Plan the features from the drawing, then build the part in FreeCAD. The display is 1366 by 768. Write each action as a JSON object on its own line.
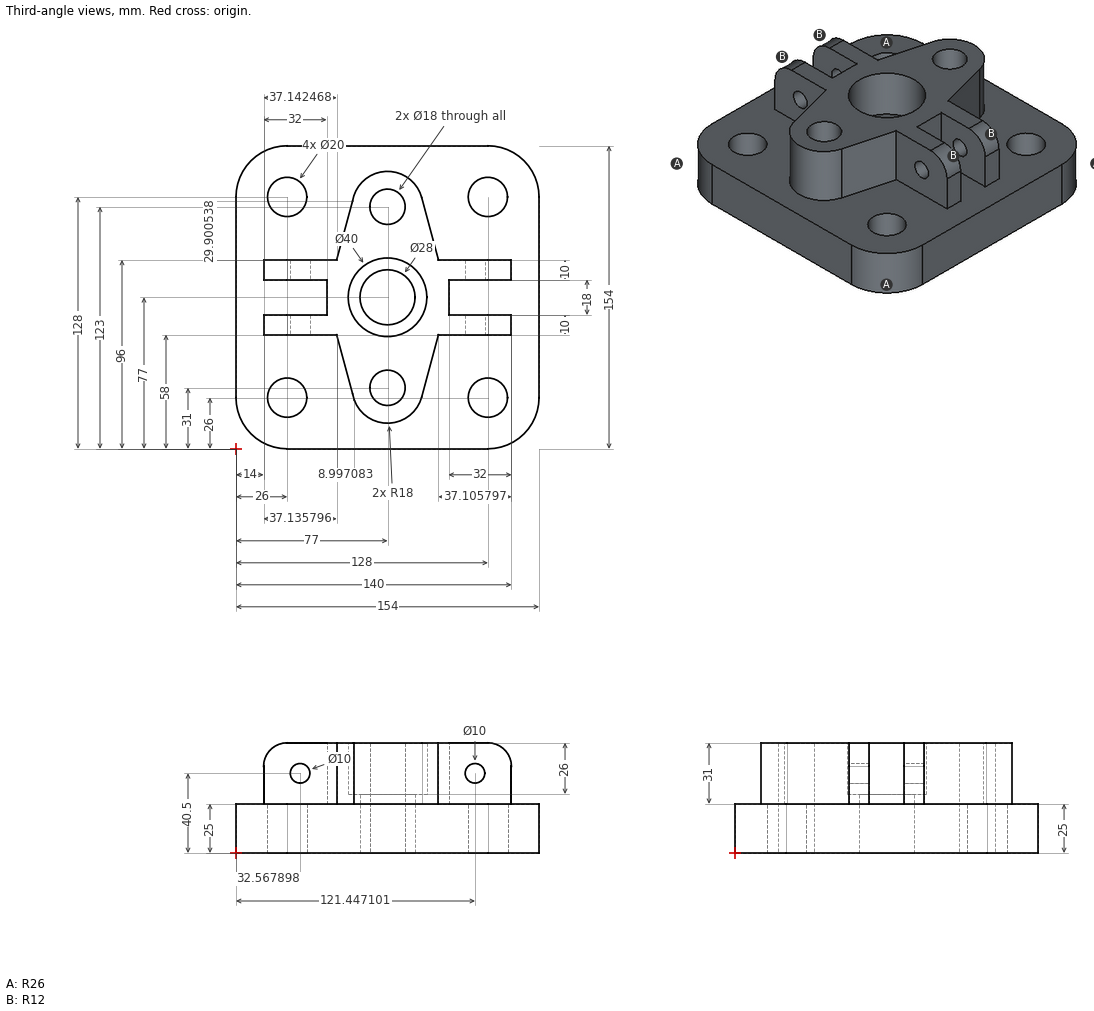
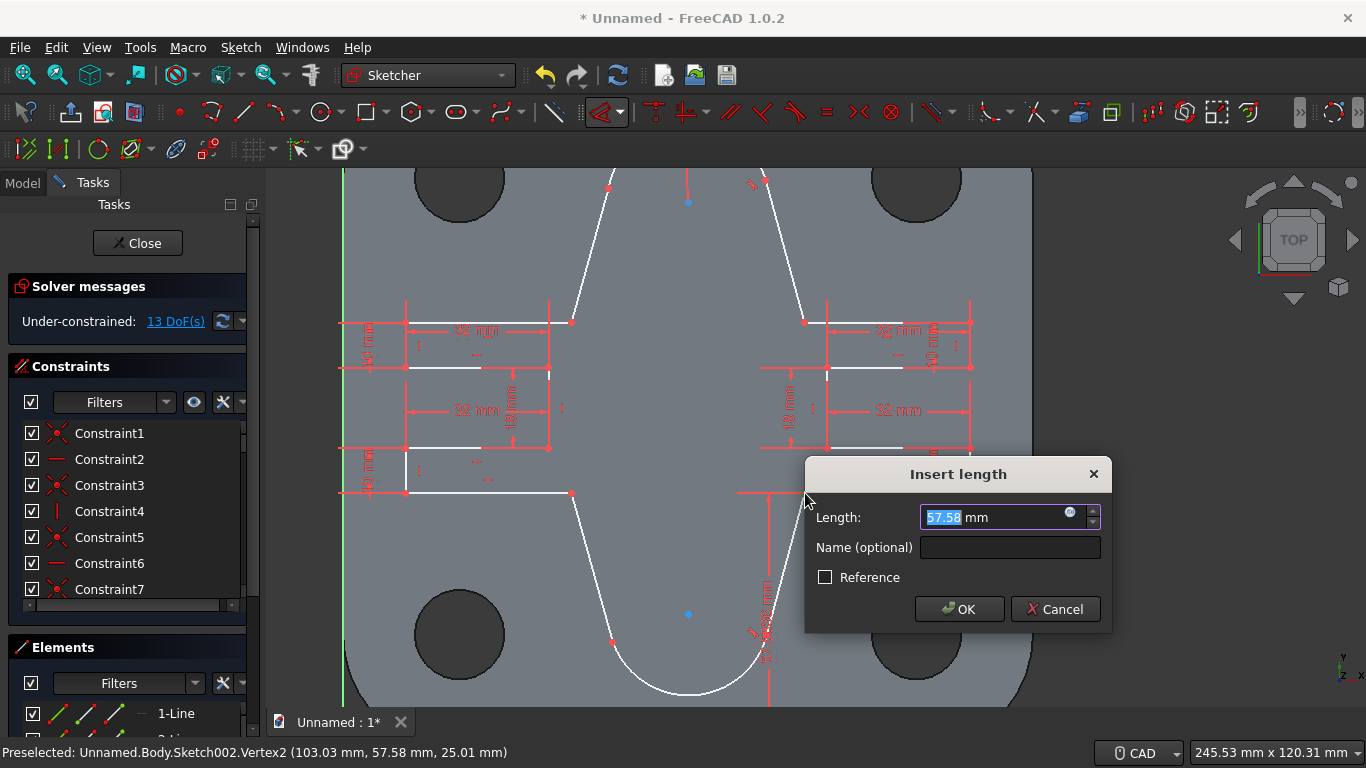
{"action": "type", "text": "58"}
{"action": "key", "text": "Return"}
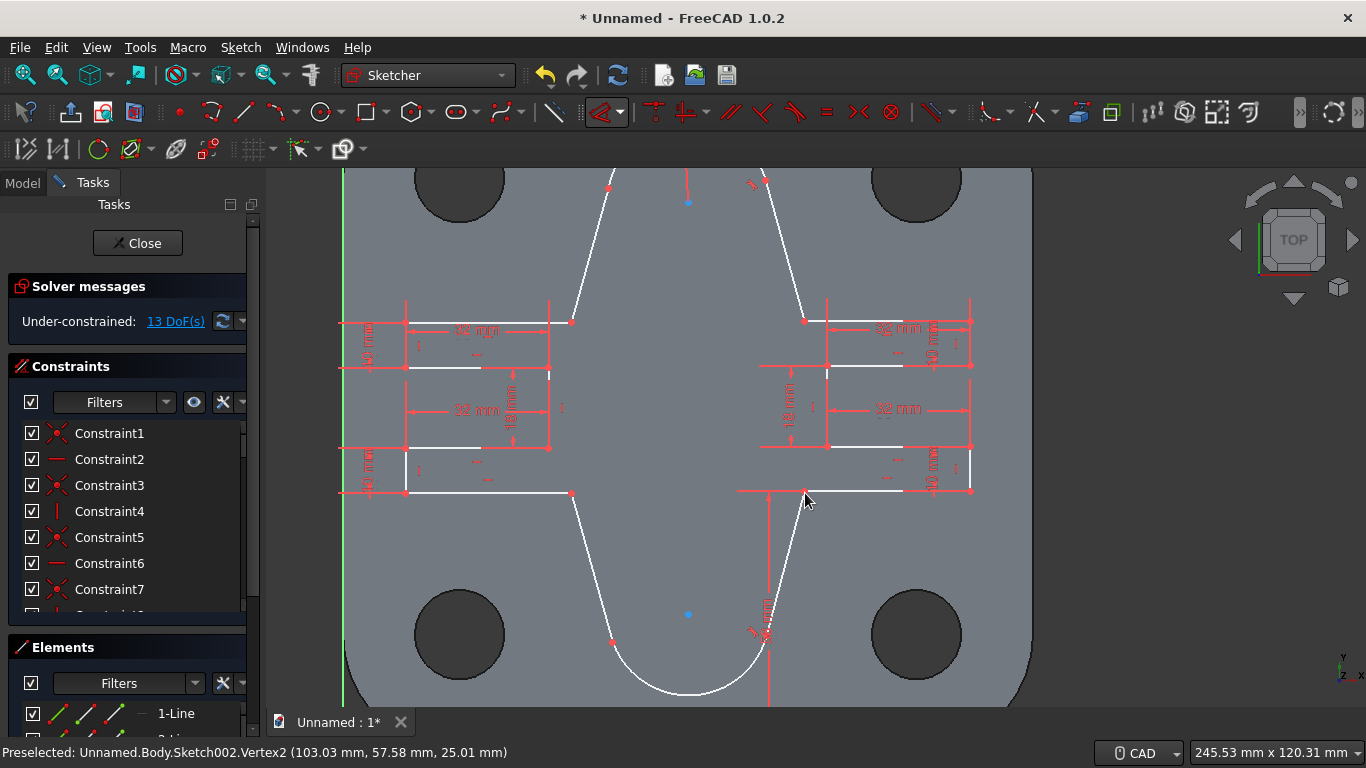
{"action": "left_click", "coordinate": [571, 323]}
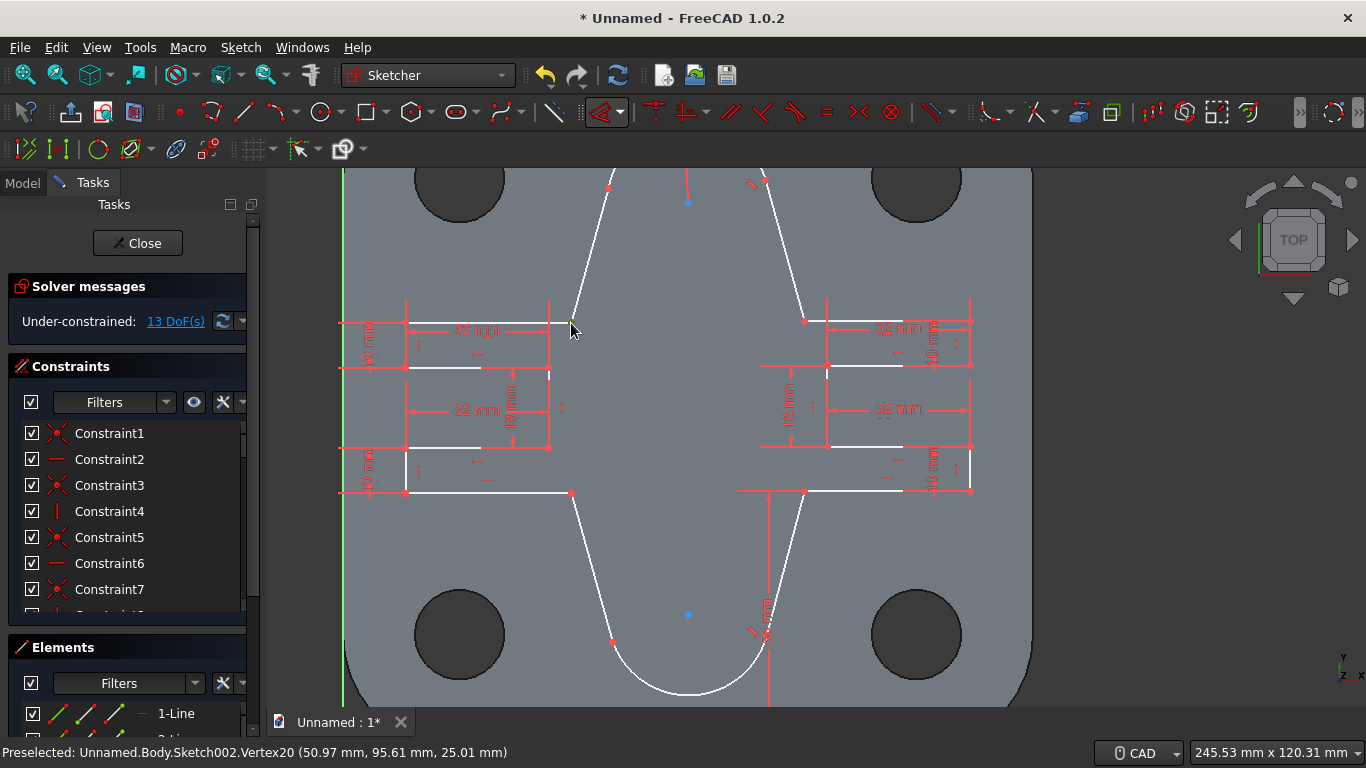
{"action": "left_click", "coordinate": [622, 112]}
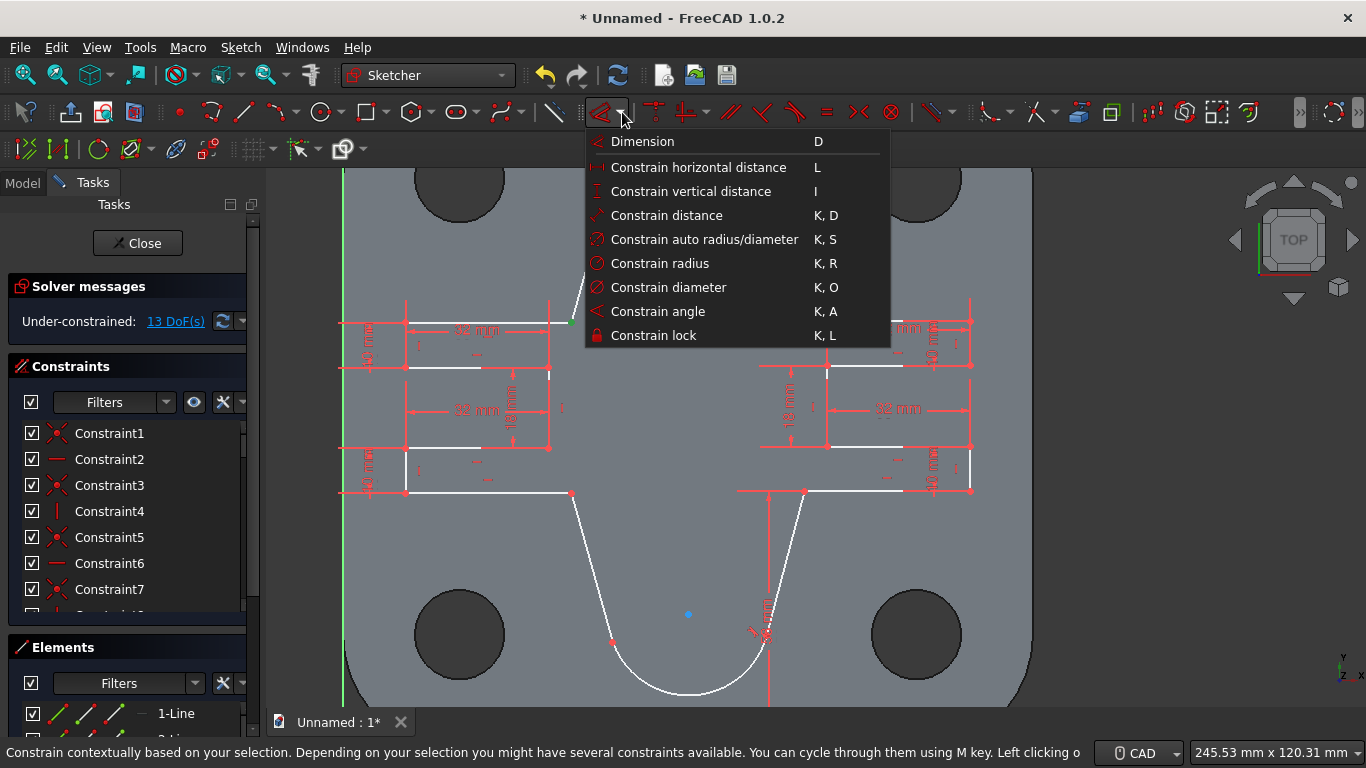
{"action": "left_click", "coordinate": [738, 191]}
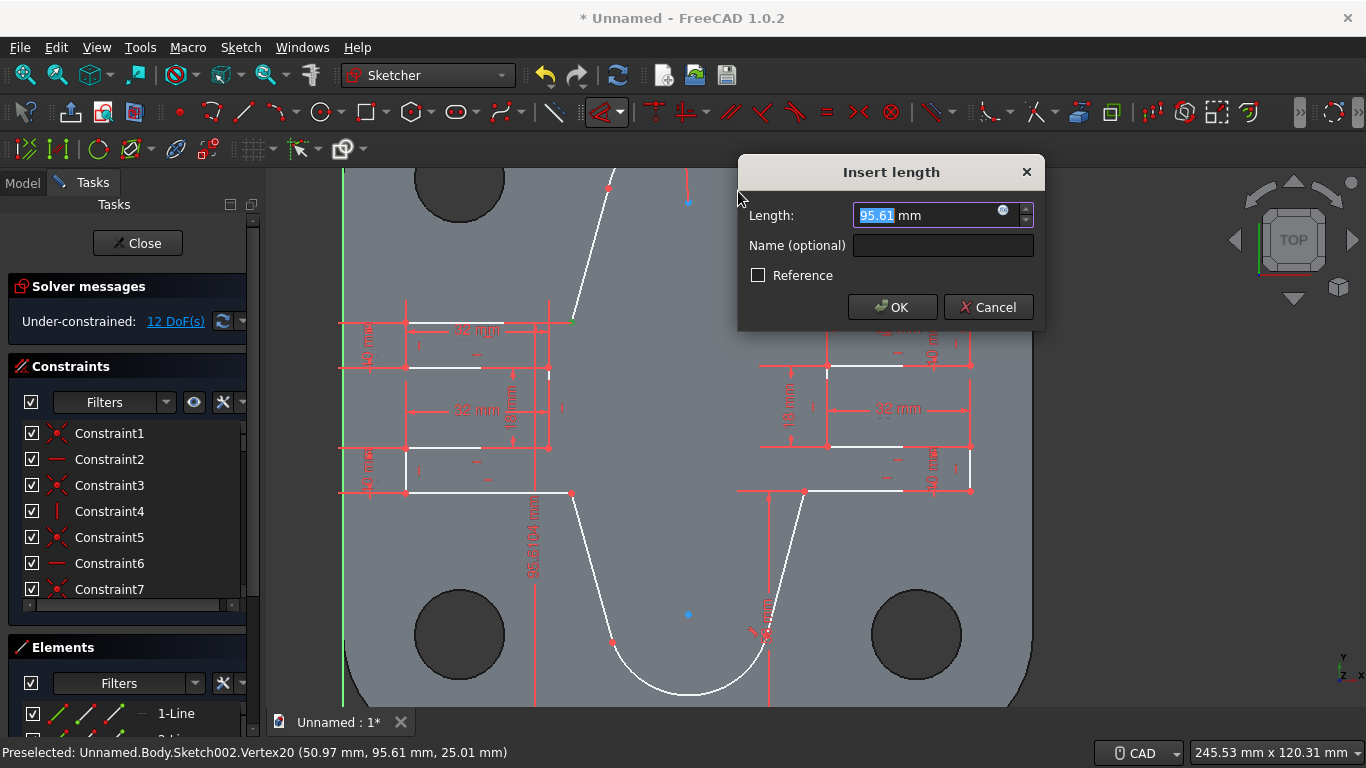
{"action": "type", "text": "96"}
{"action": "key", "text": "Return"}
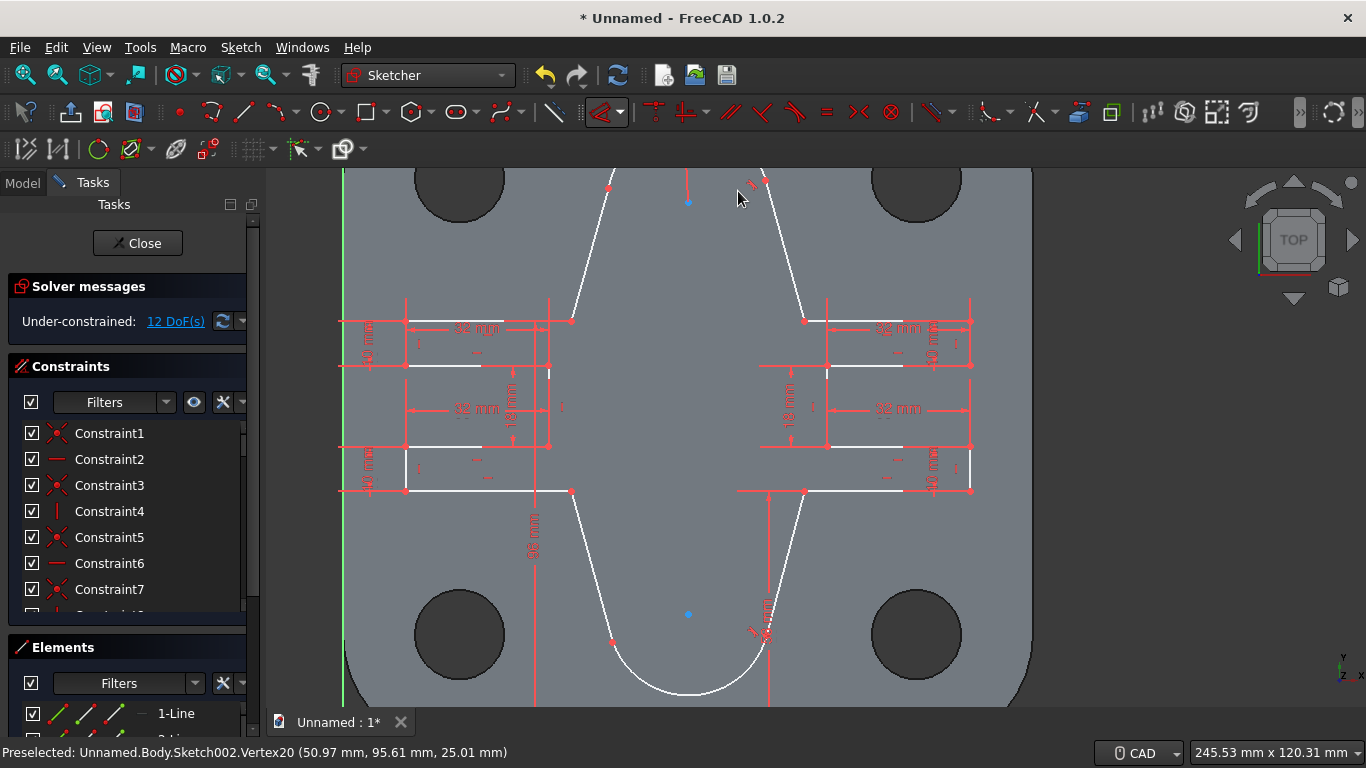
{"action": "left_click", "coordinate": [406, 321]}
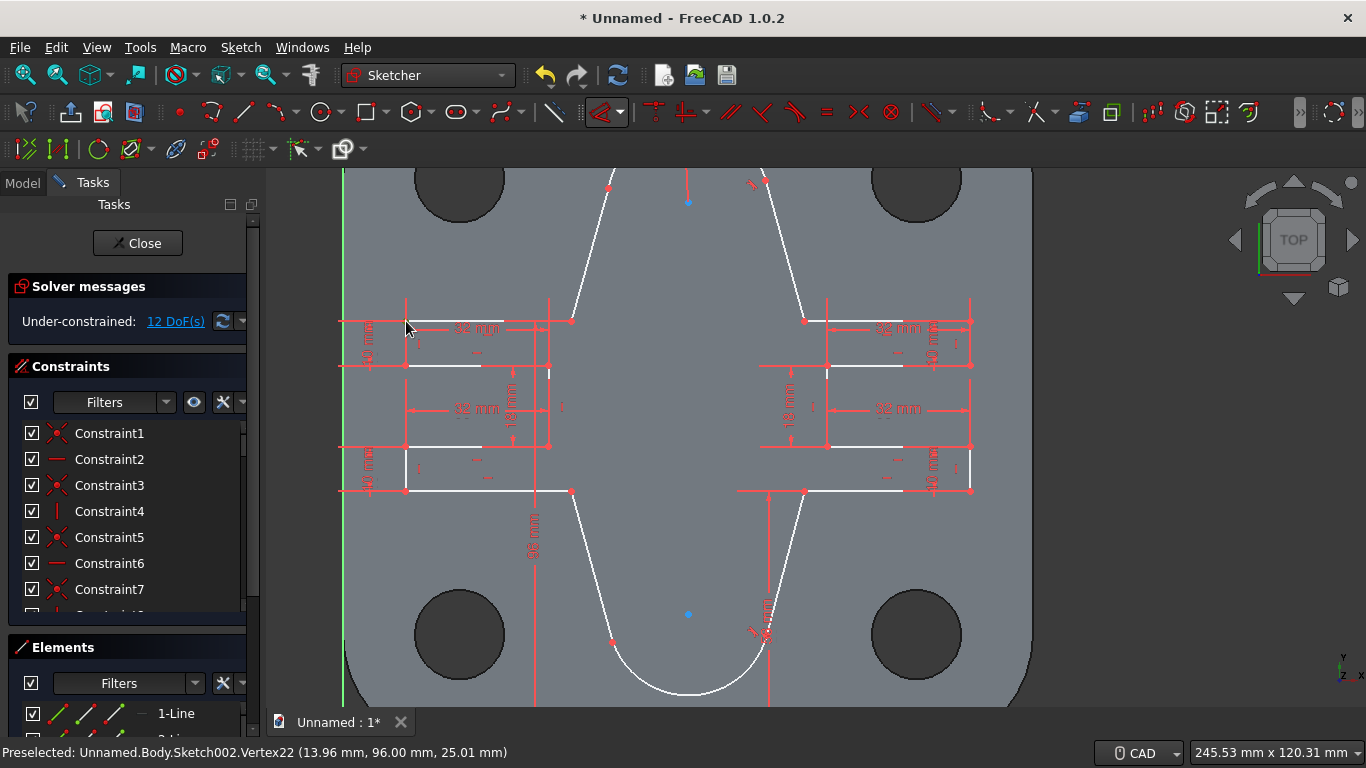
{"action": "left_click", "coordinate": [622, 112]}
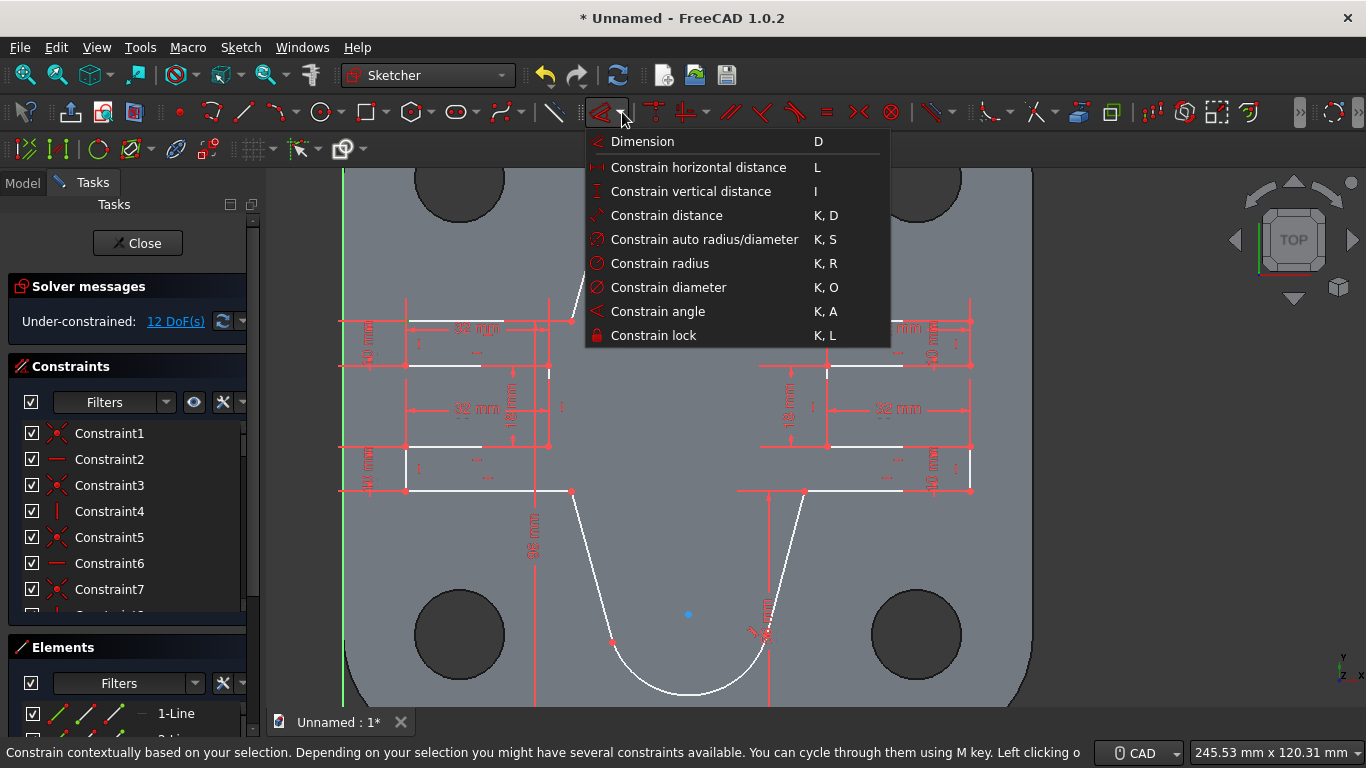
{"action": "left_click", "coordinate": [738, 167]}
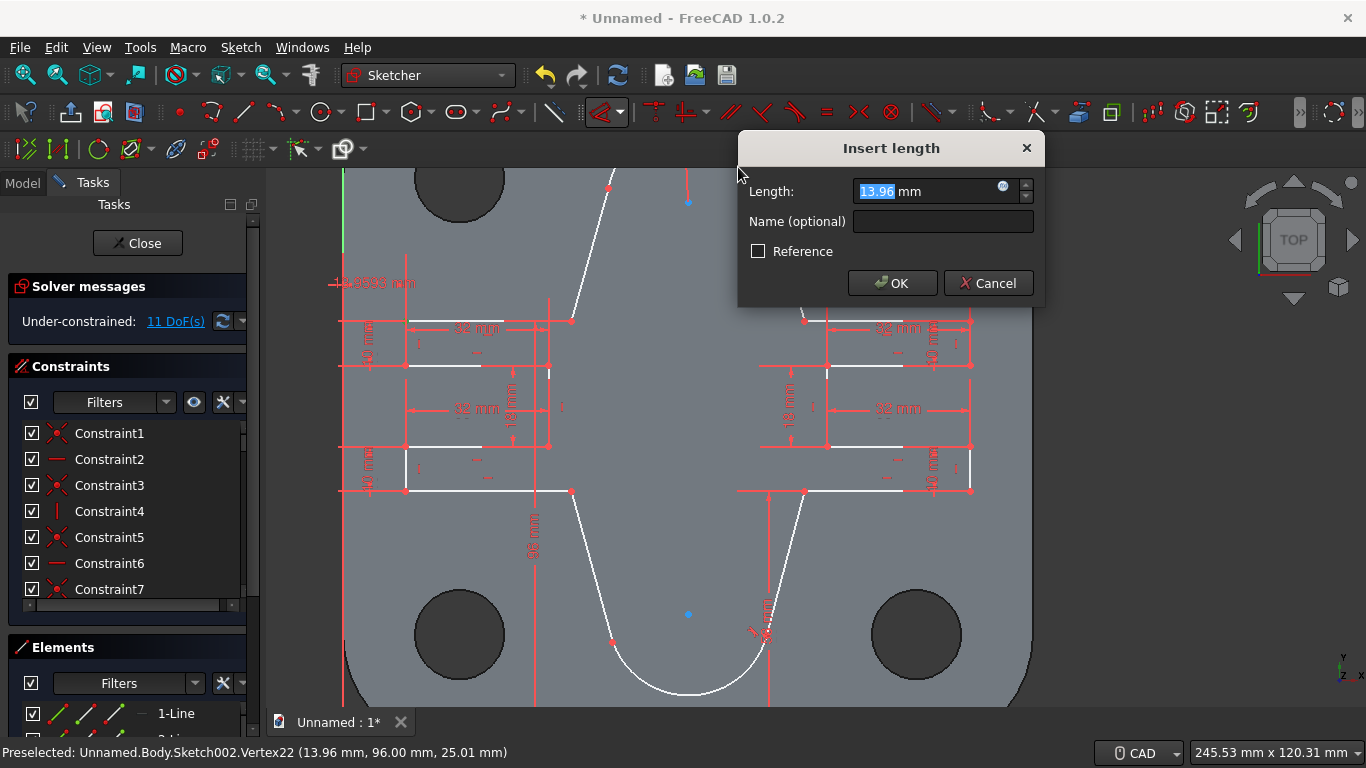
{"action": "type", "text": "14"}
{"action": "key", "text": "Return"}